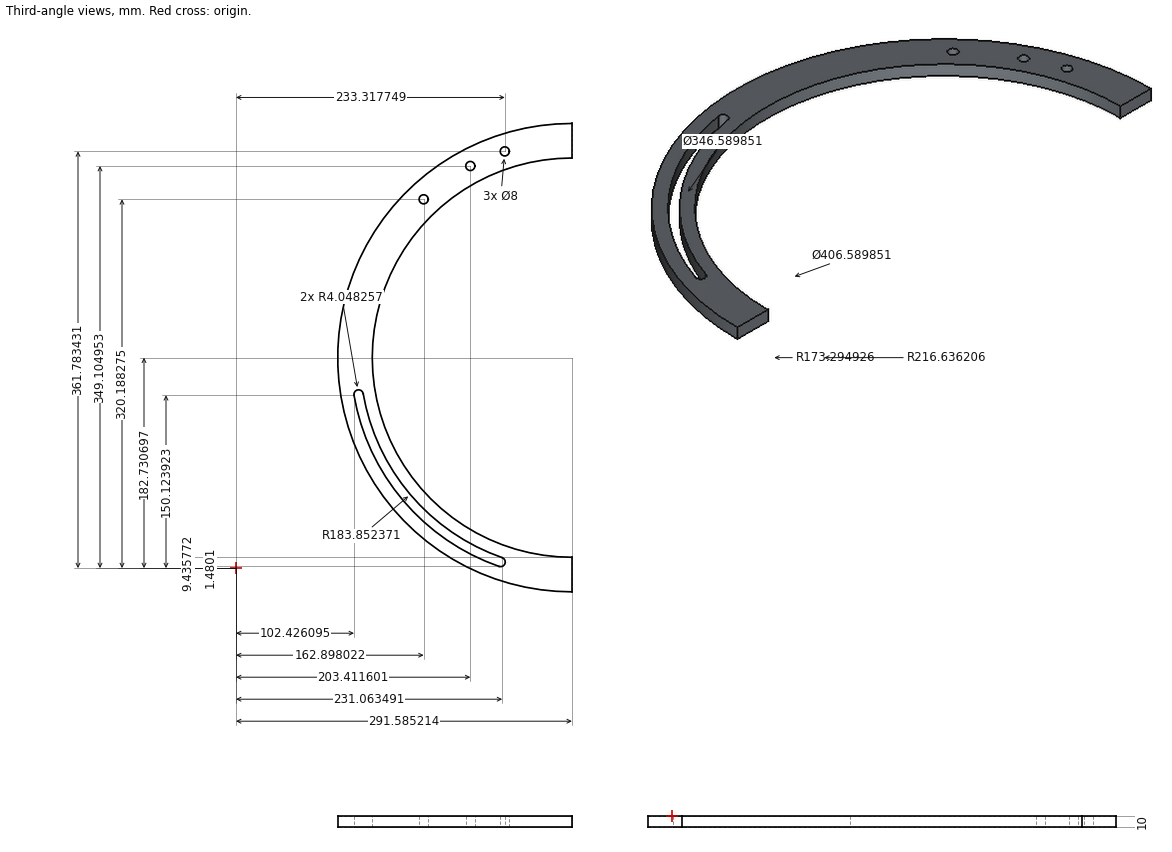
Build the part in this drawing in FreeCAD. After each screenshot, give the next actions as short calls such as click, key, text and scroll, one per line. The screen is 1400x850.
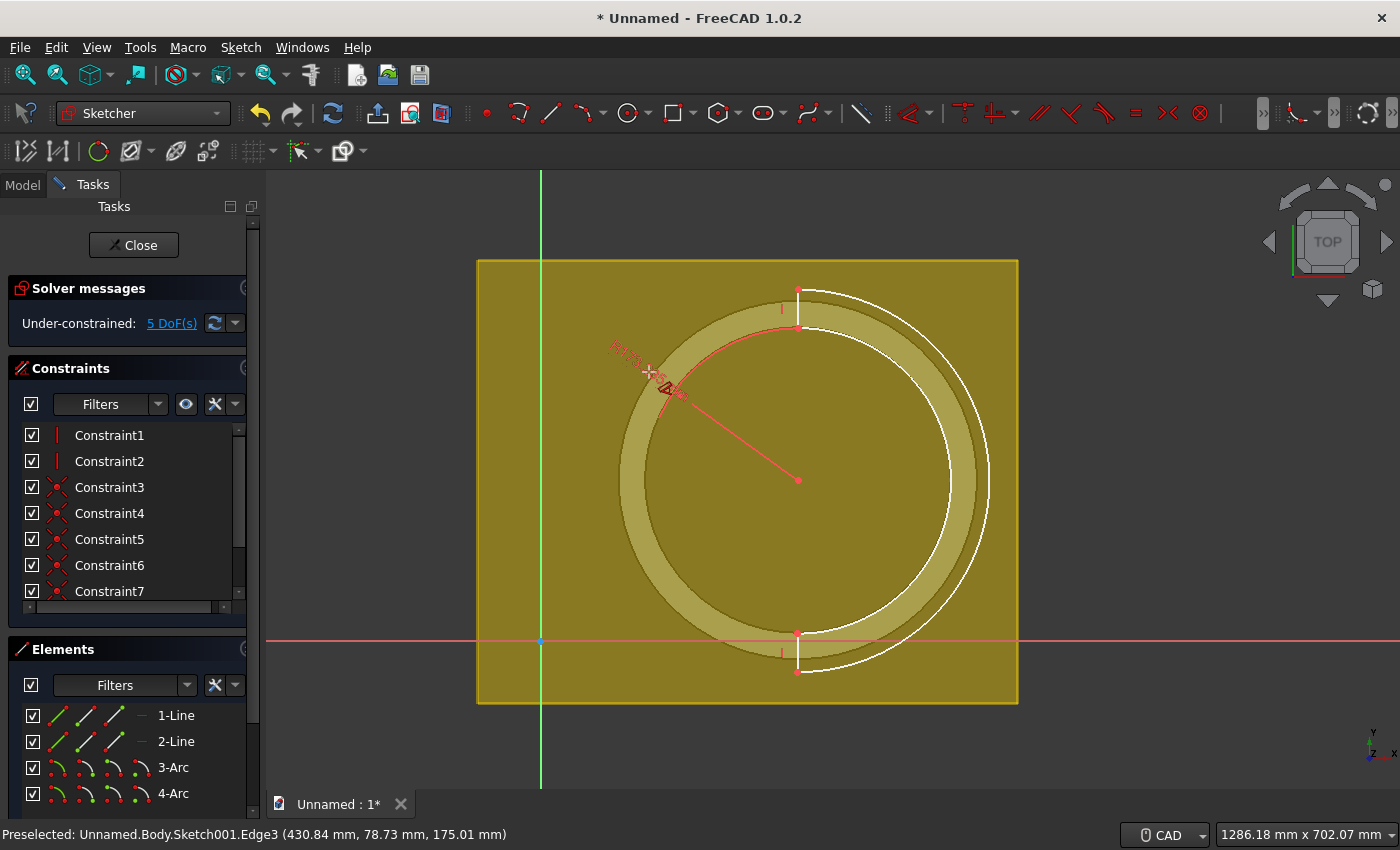
click(953, 593)
click(979, 612)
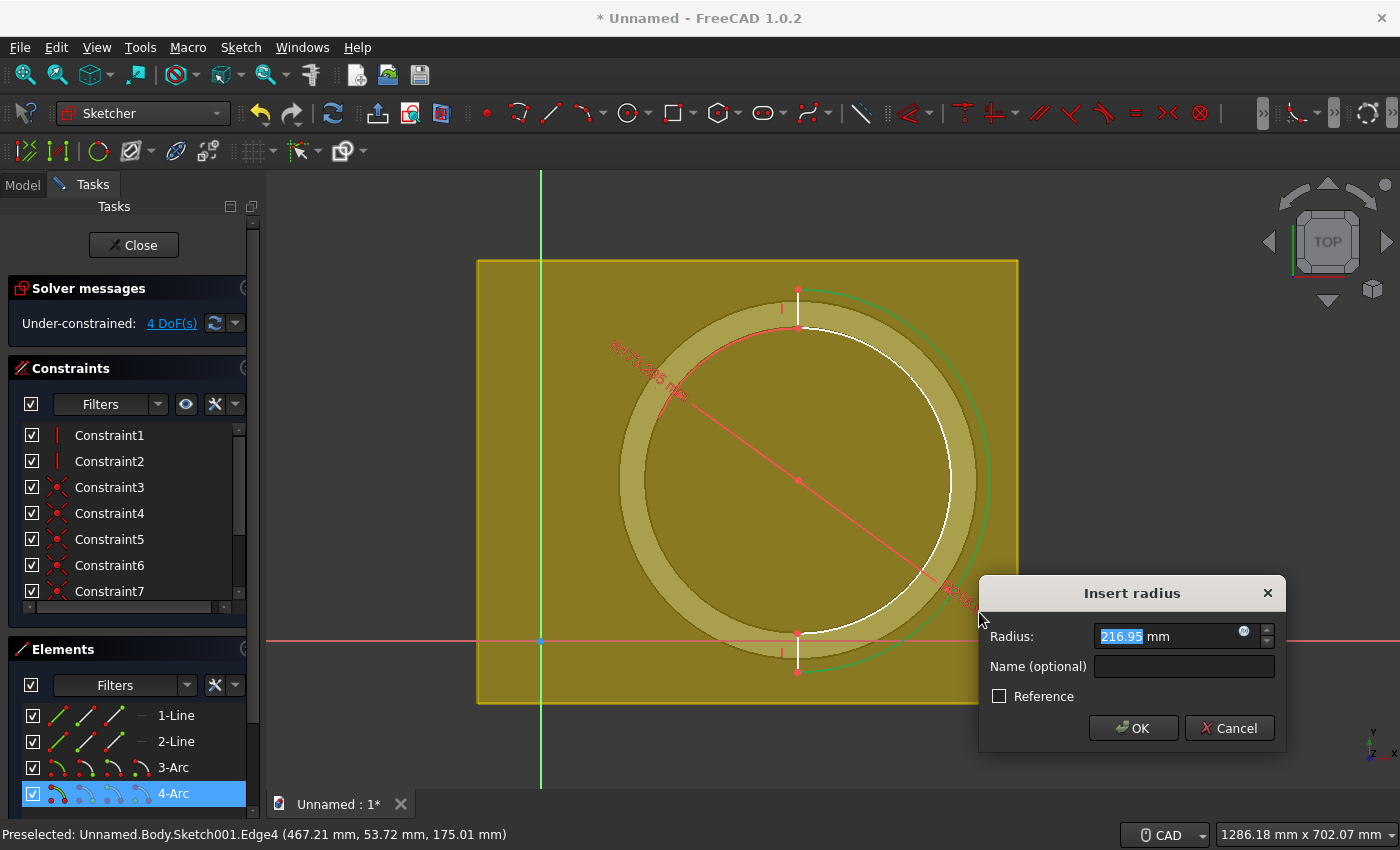
text(216.636206)
key(Return)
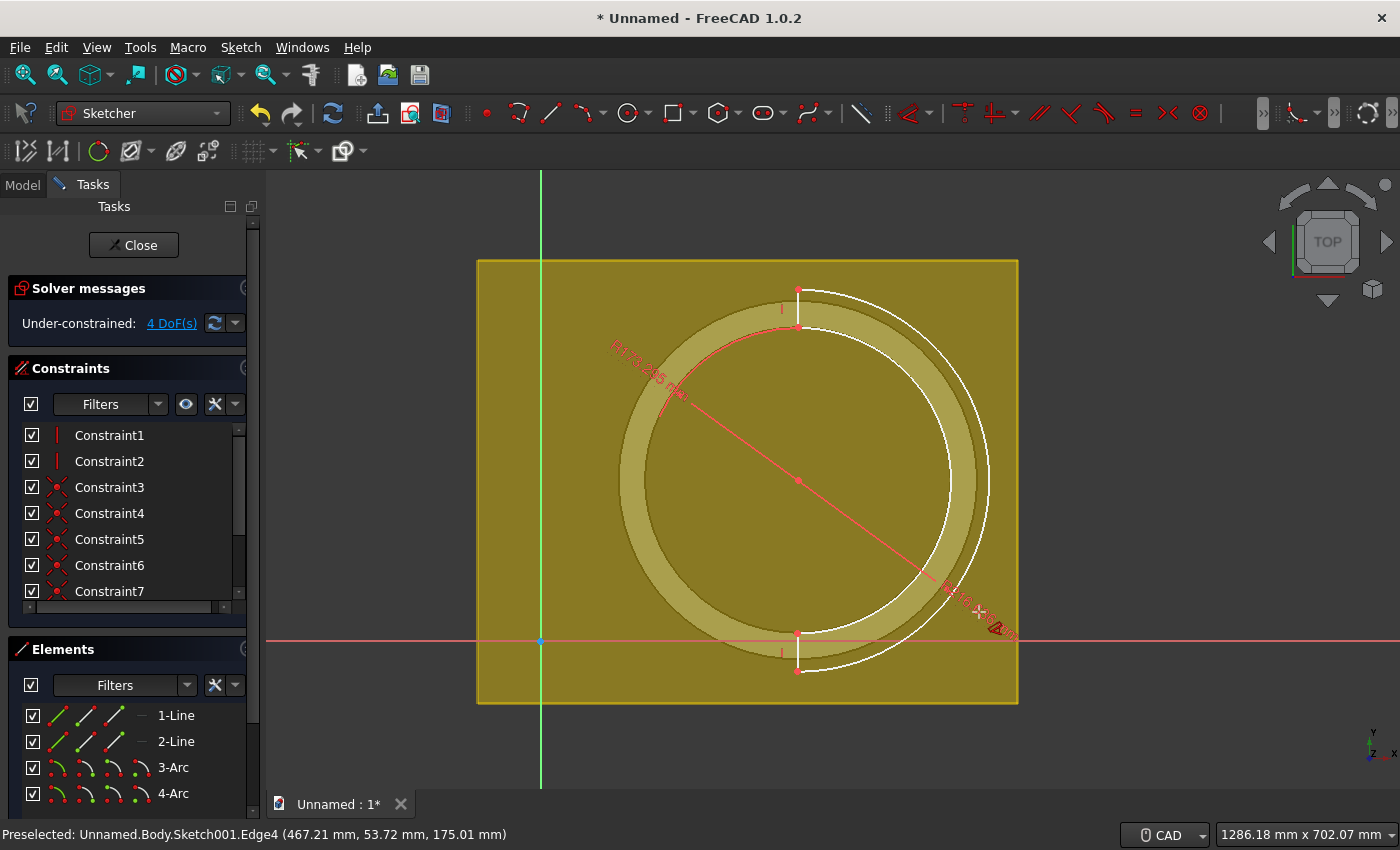
scroll(798, 634, up, 8)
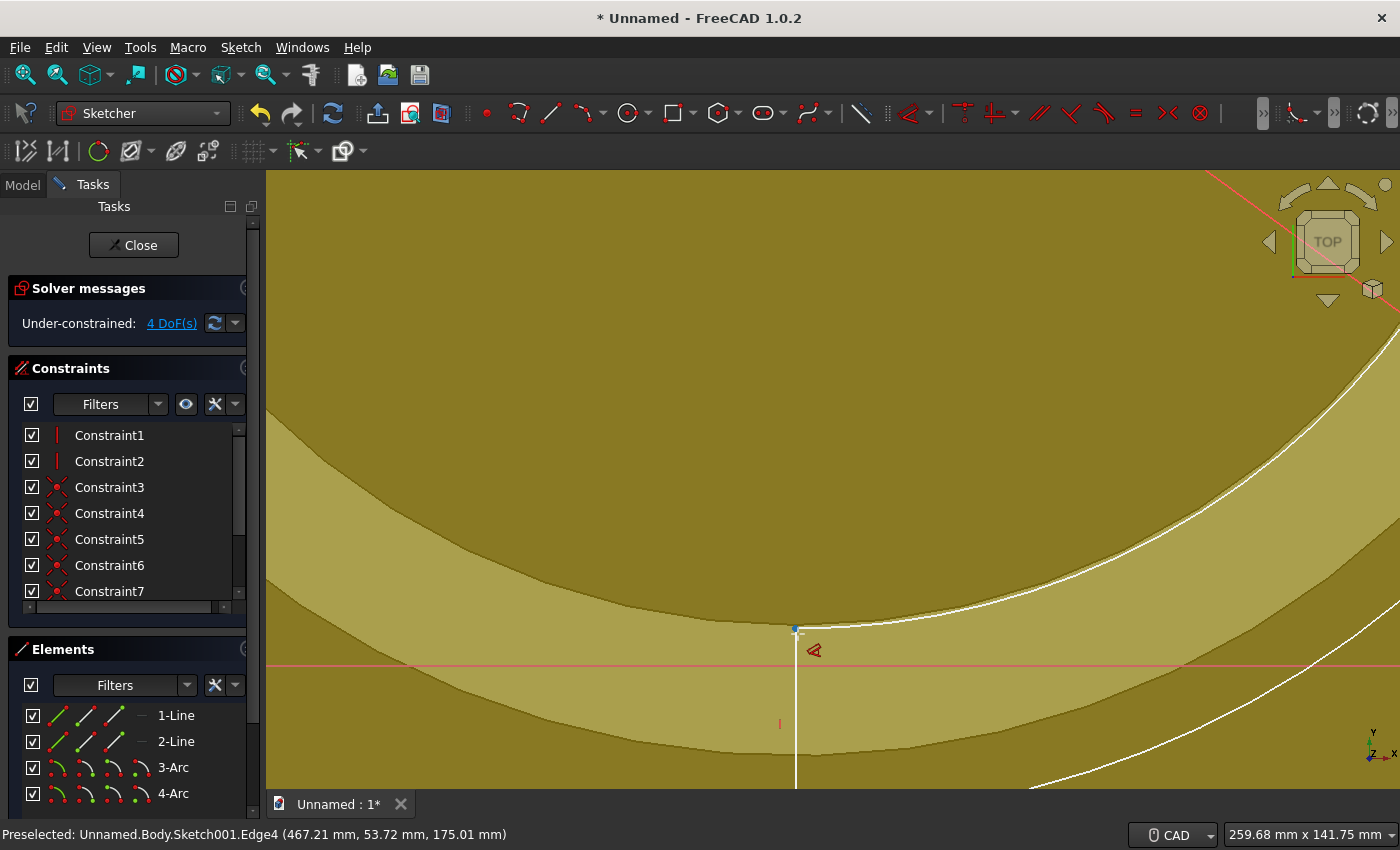
click(796, 629)
click(830, 647)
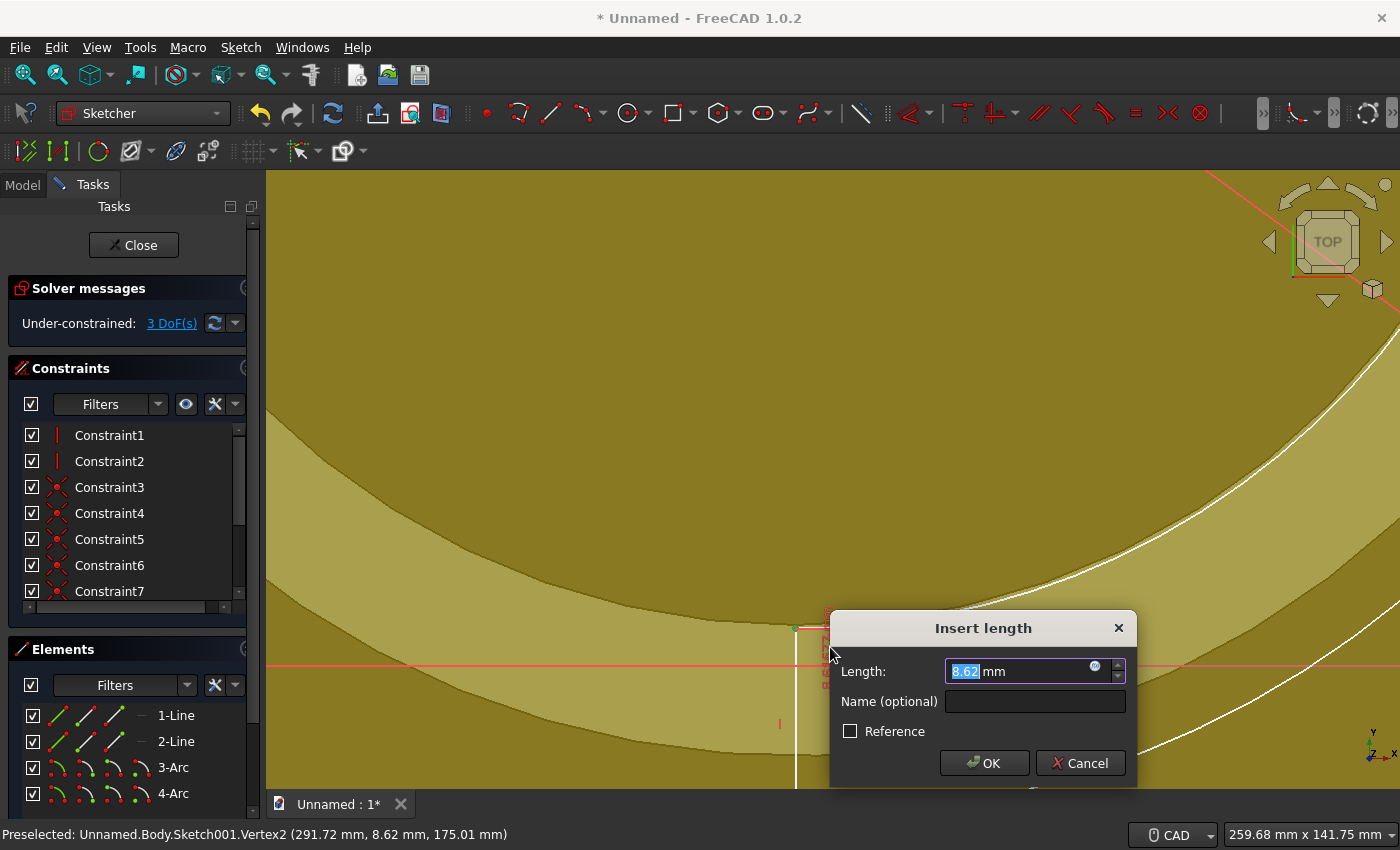
text(9.435772)
key(Return)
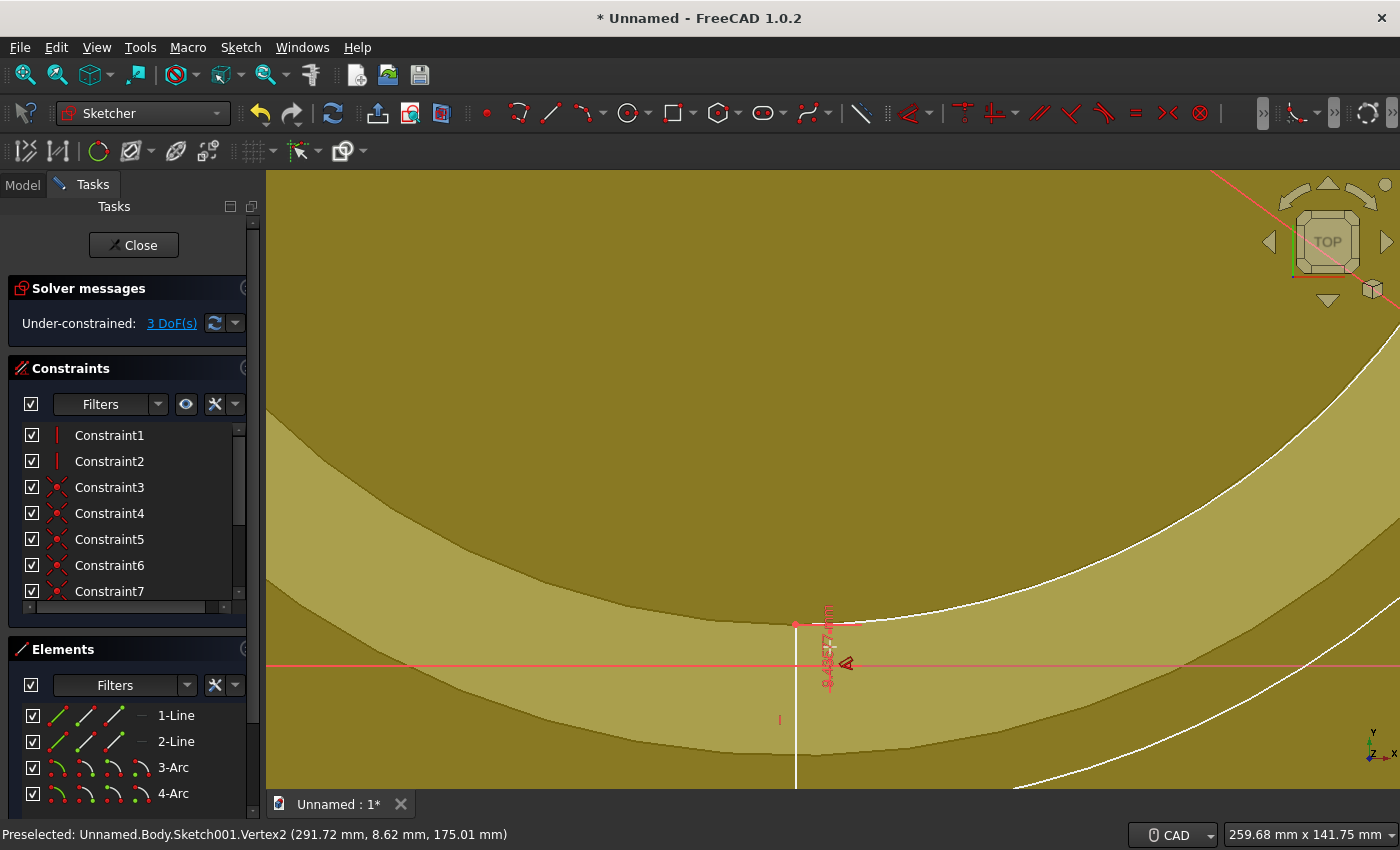
scroll(798, 634, down, 8)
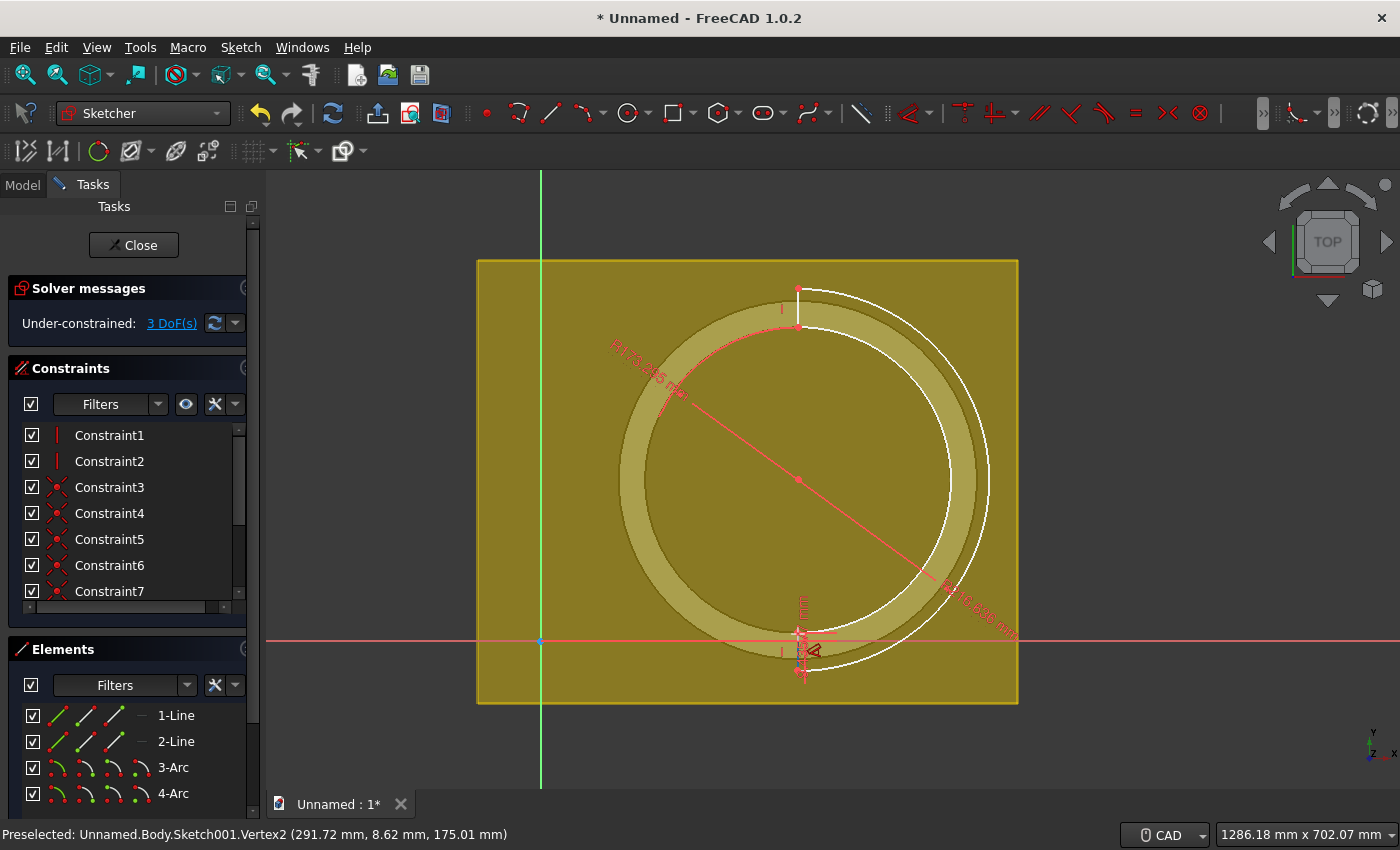
click(798, 671)
click(669, 705)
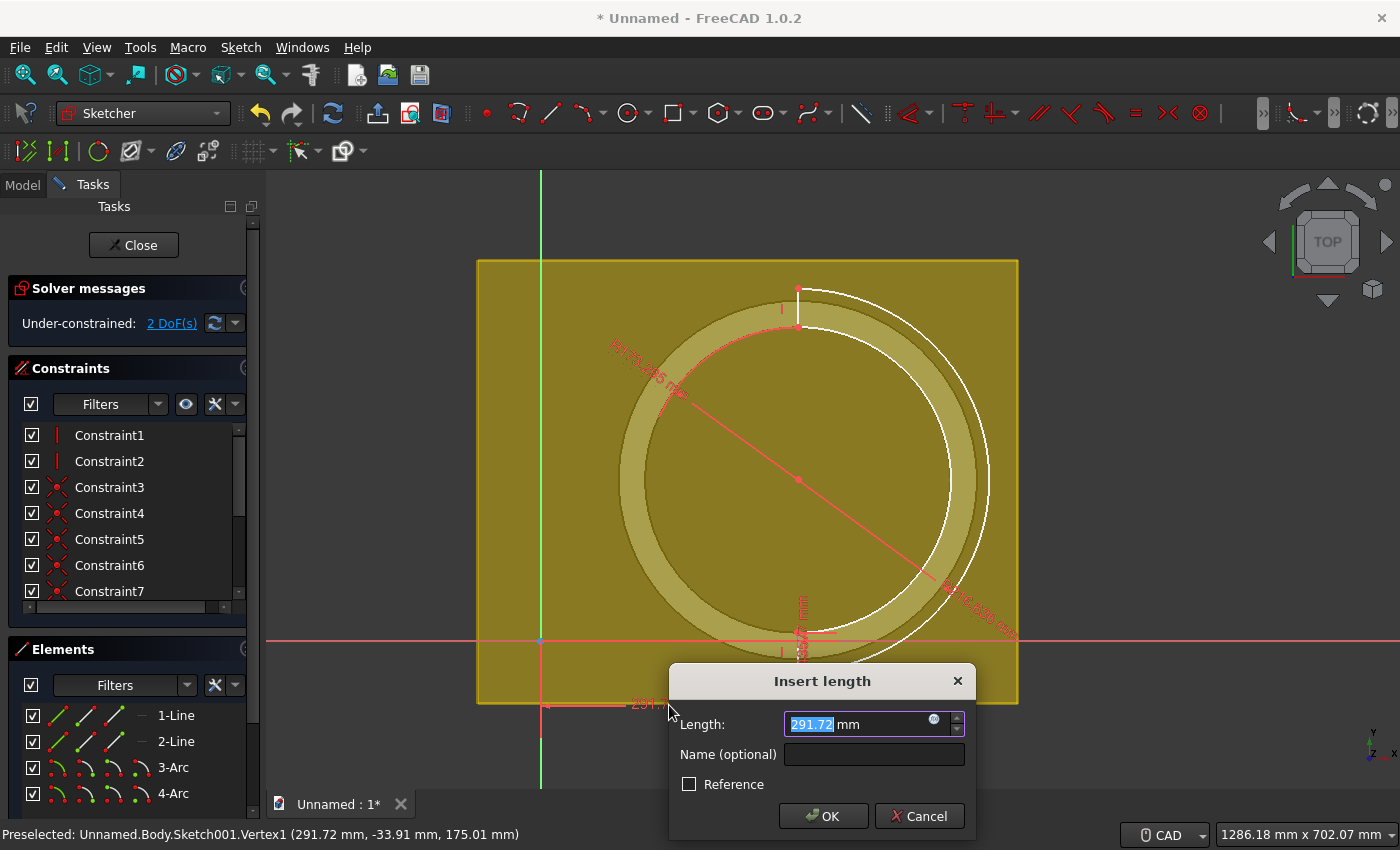
text(291.585214)
key(Return)